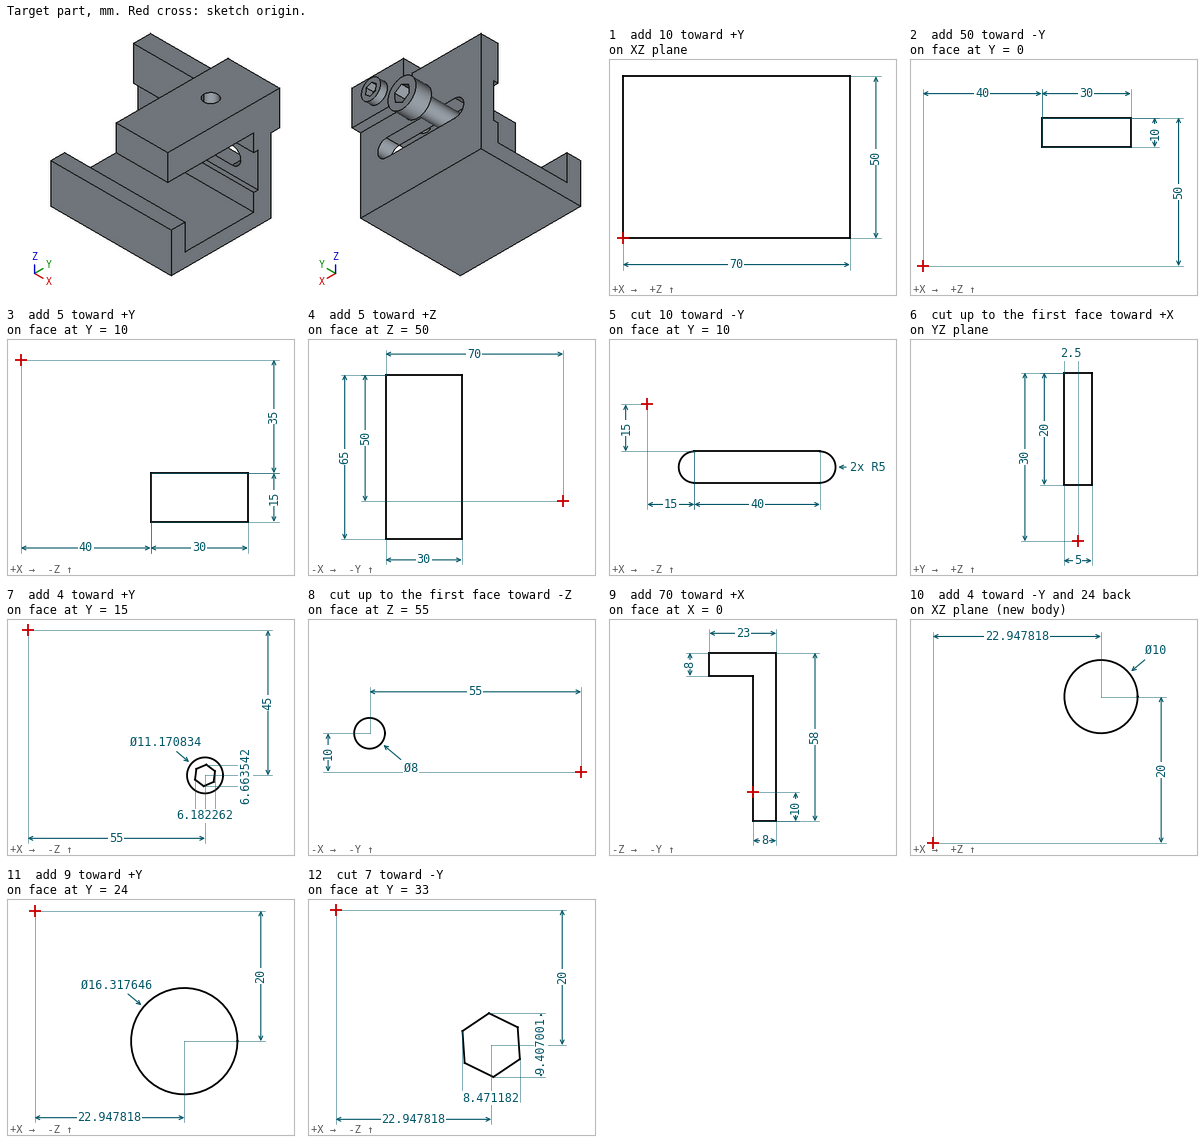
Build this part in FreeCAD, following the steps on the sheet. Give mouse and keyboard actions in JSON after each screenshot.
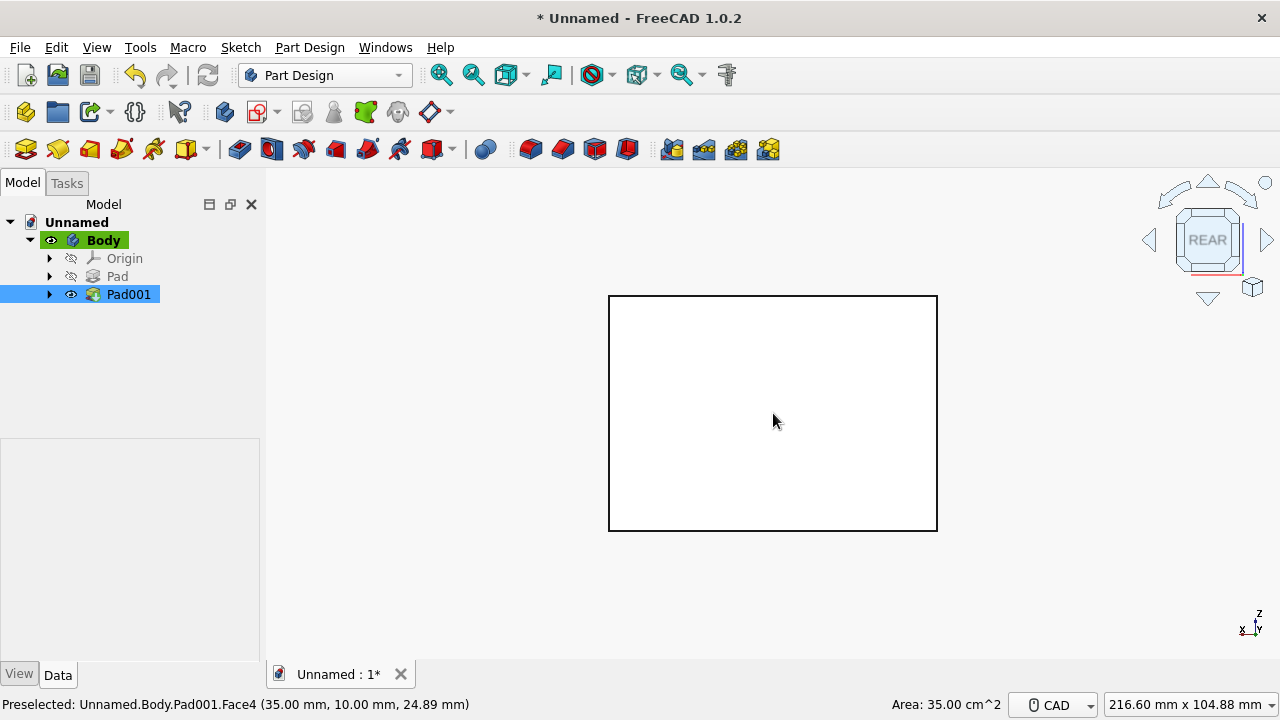
{"action": "left_click", "coordinate": [258, 112]}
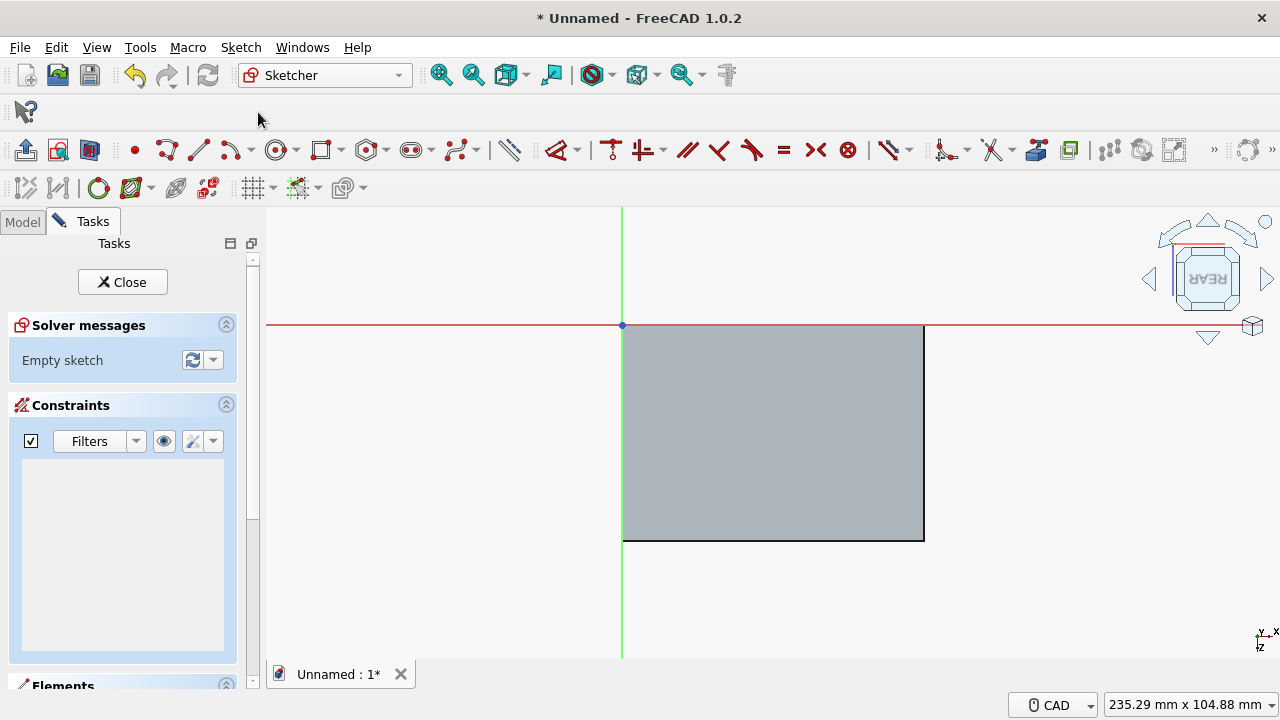
{"action": "left_click", "coordinate": [322, 150]}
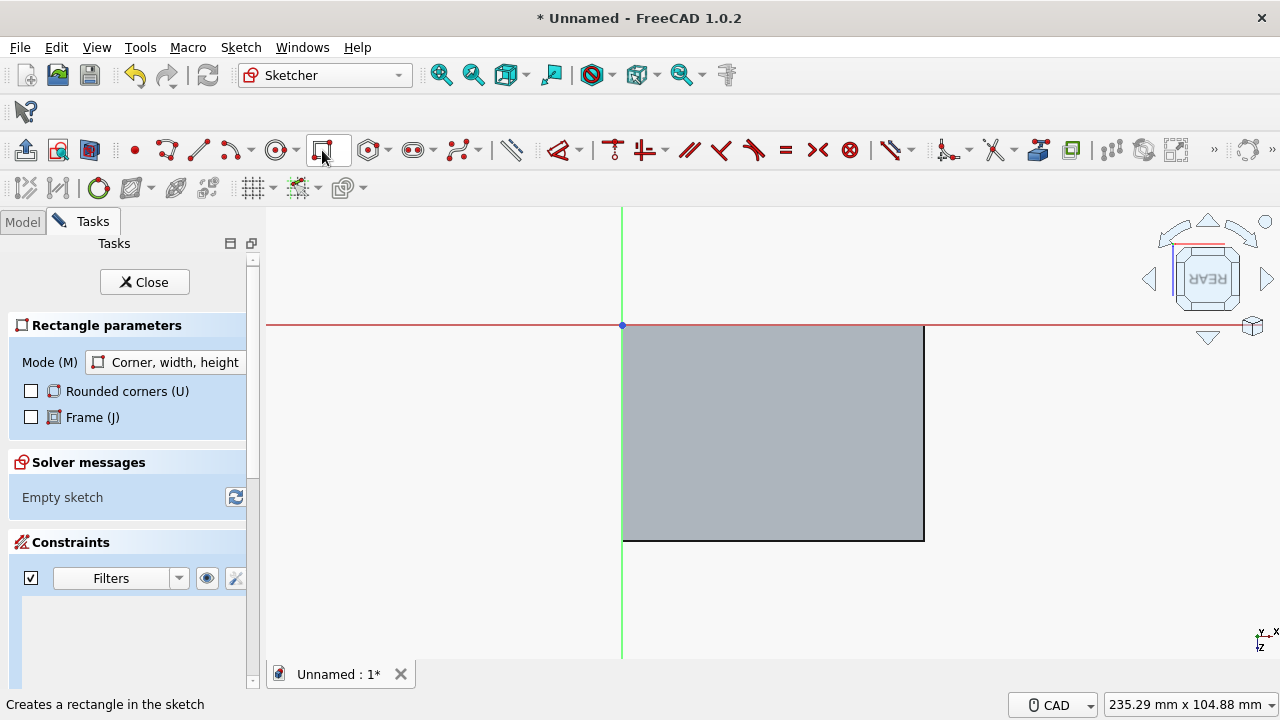
{"action": "left_click", "coordinate": [795, 476]}
{"action": "left_click", "coordinate": [924, 541]}
{"action": "key", "text": "Escape"}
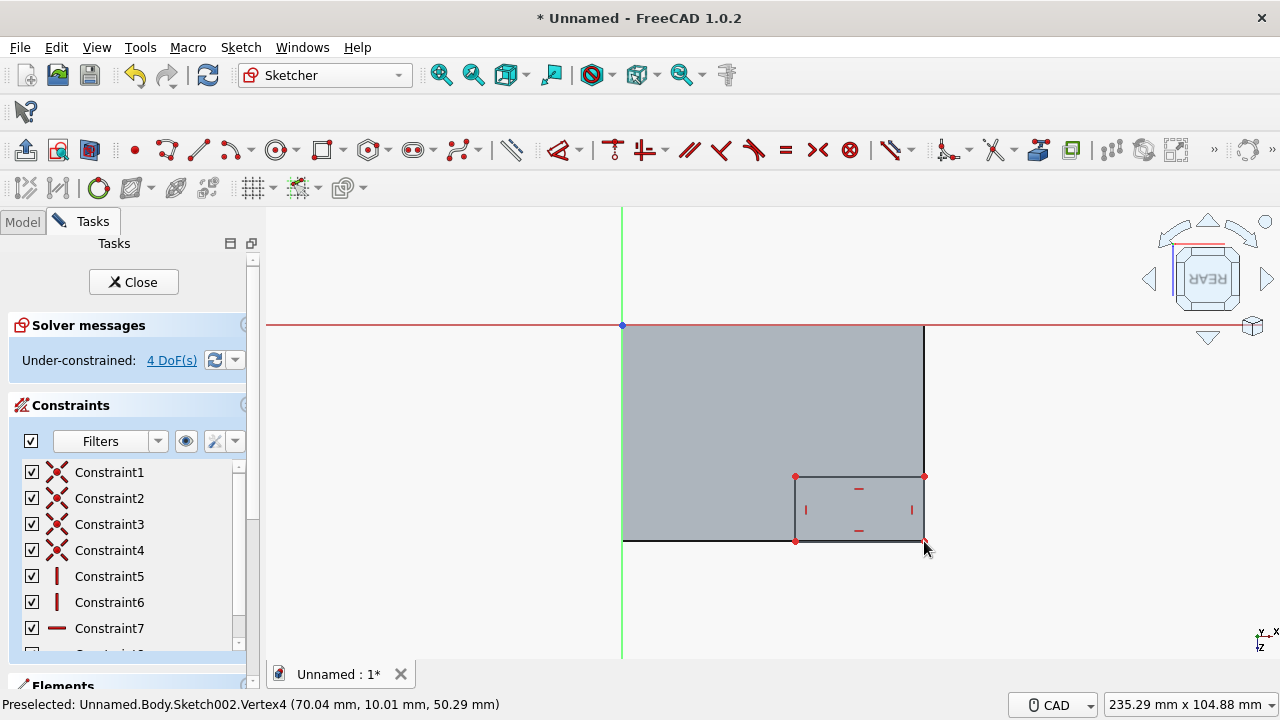
{"action": "left_click", "coordinate": [558, 150]}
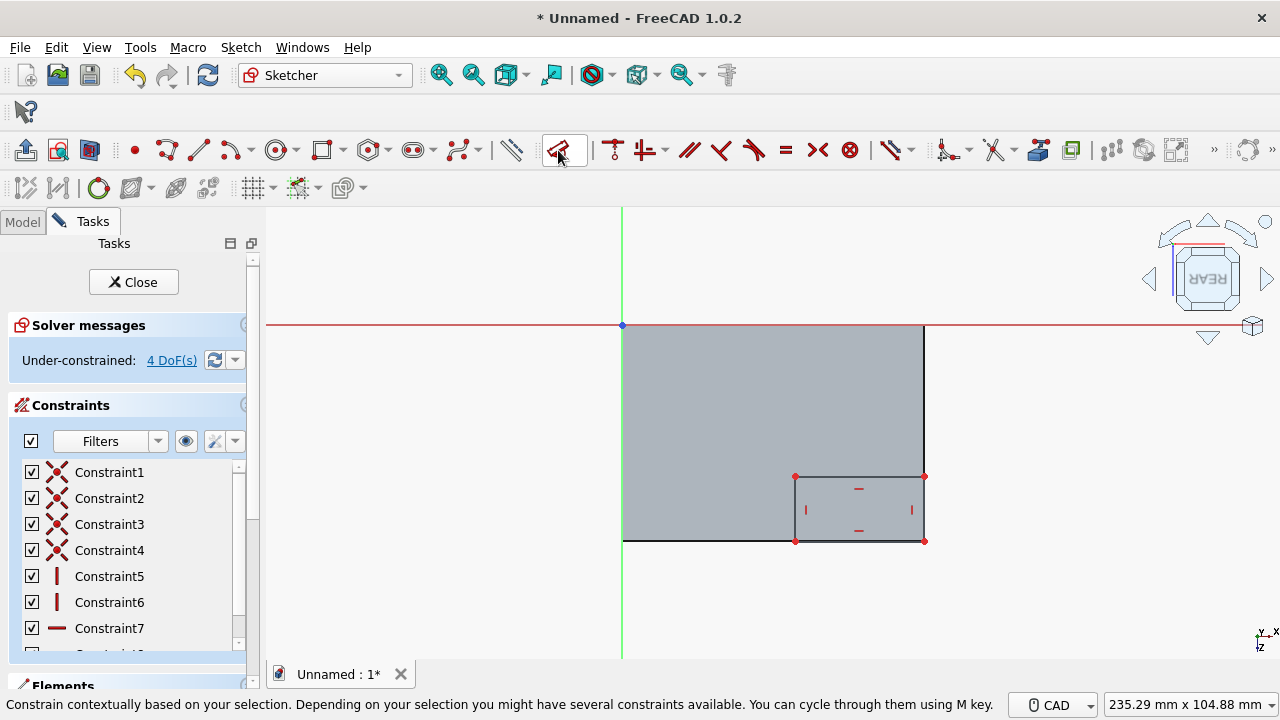
{"action": "left_click", "coordinate": [795, 497]}
{"action": "left_click", "coordinate": [829, 510]}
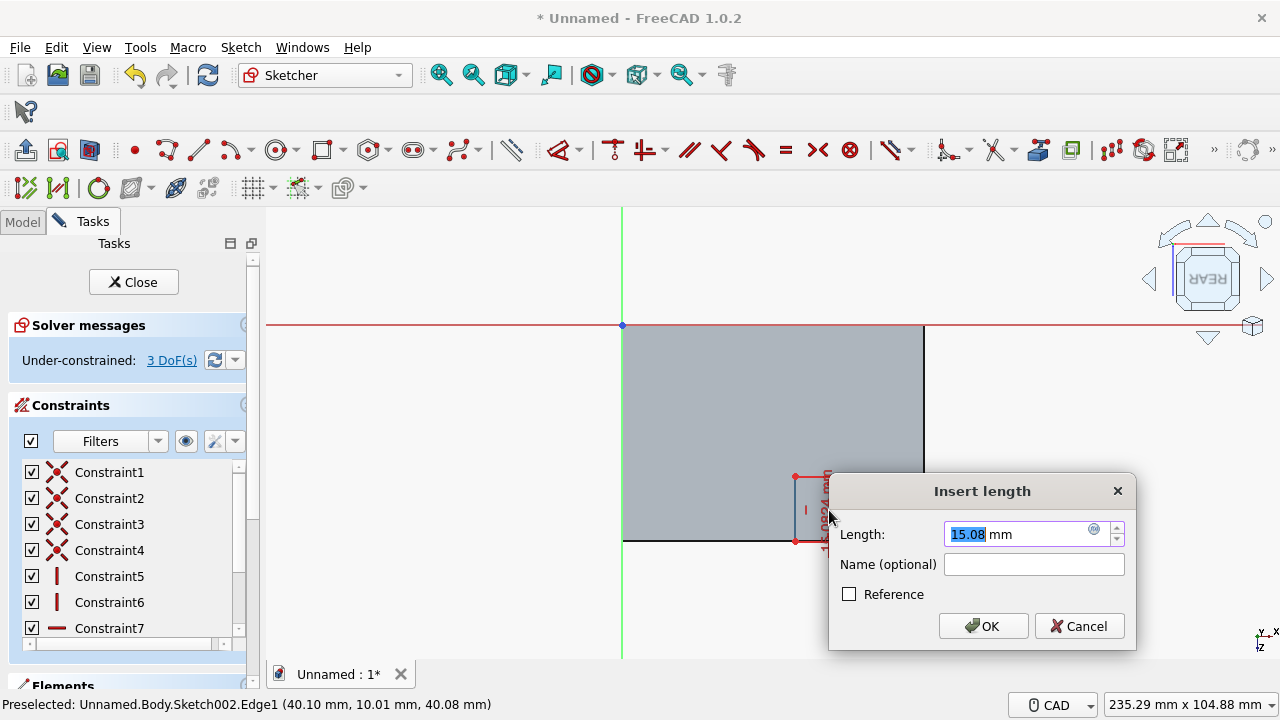
{"action": "type", "text": "15"}
{"action": "key", "text": "Return"}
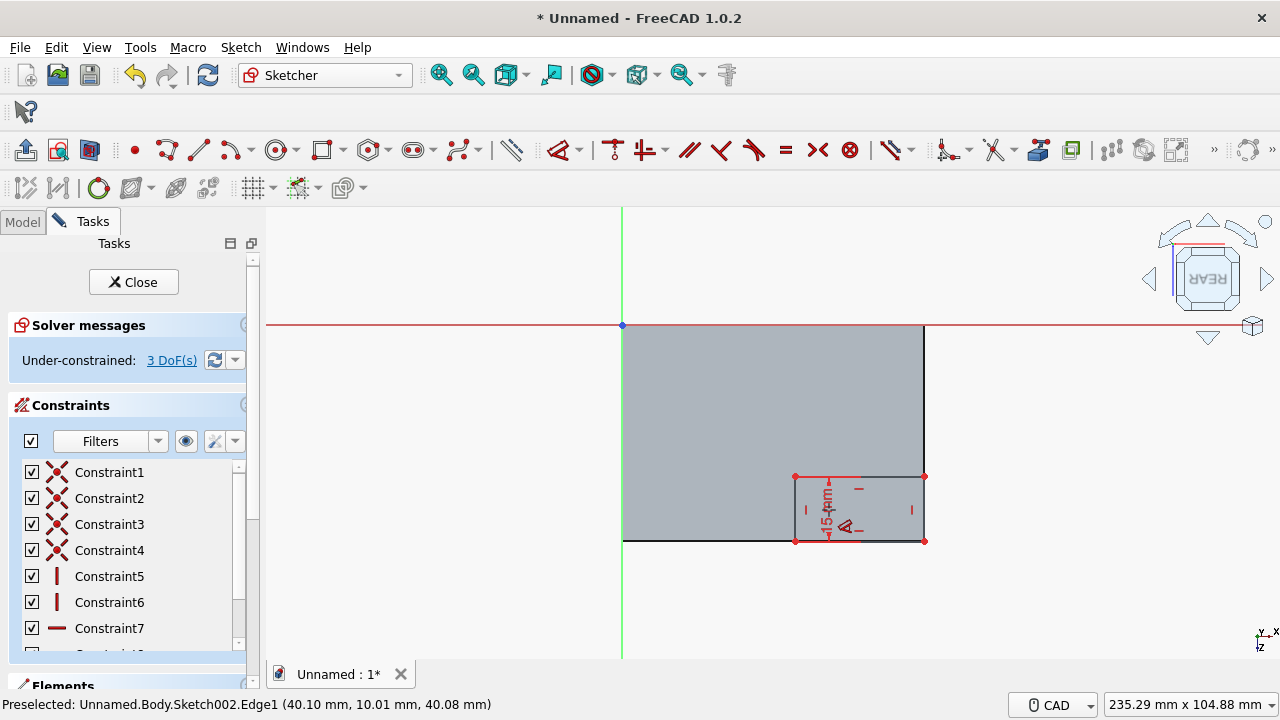
{"action": "left_click", "coordinate": [834, 542]}
{"action": "left_click", "coordinate": [860, 576]}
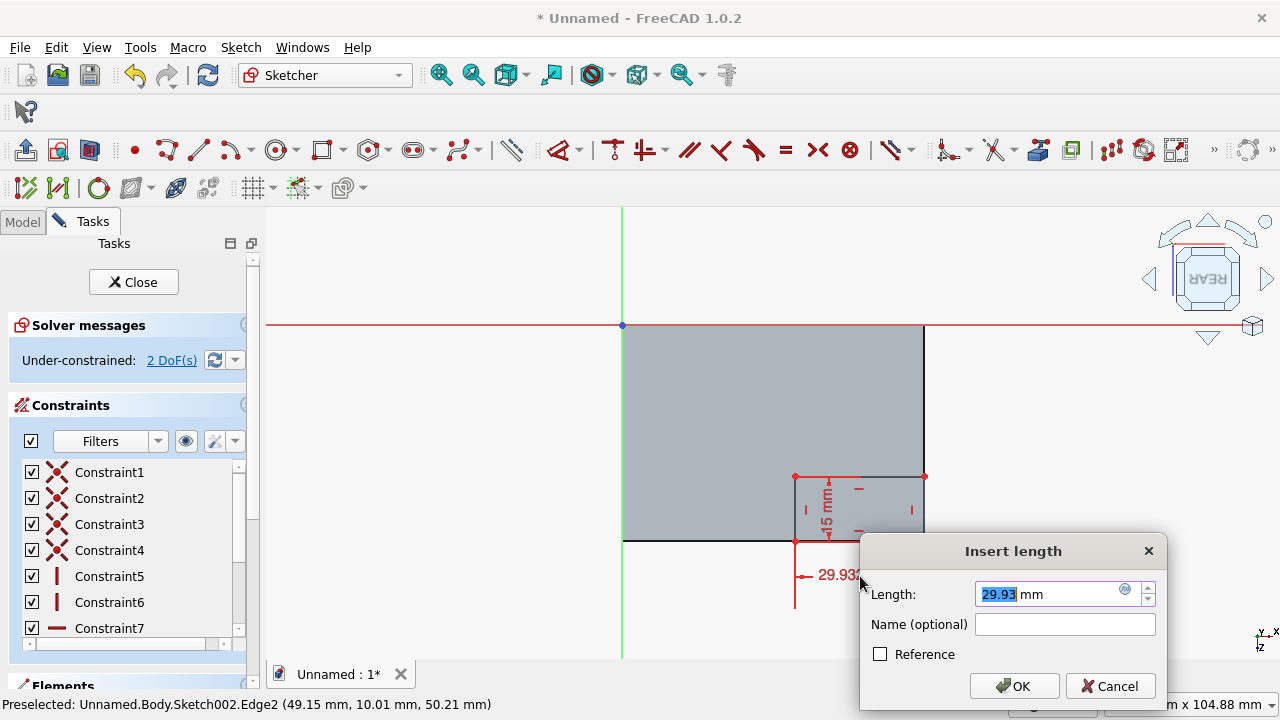
{"action": "type", "text": "30"}
{"action": "key", "text": "Return"}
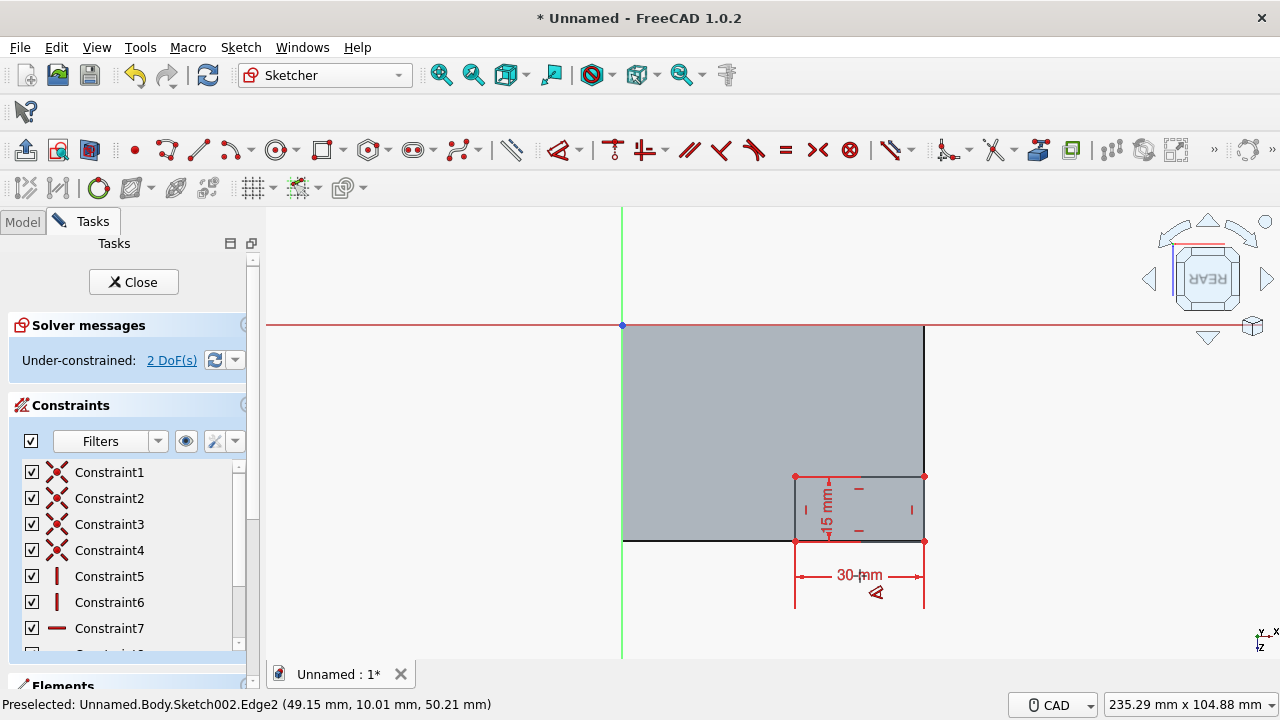
{"action": "left_click", "coordinate": [795, 477]}
{"action": "left_click", "coordinate": [709, 291]}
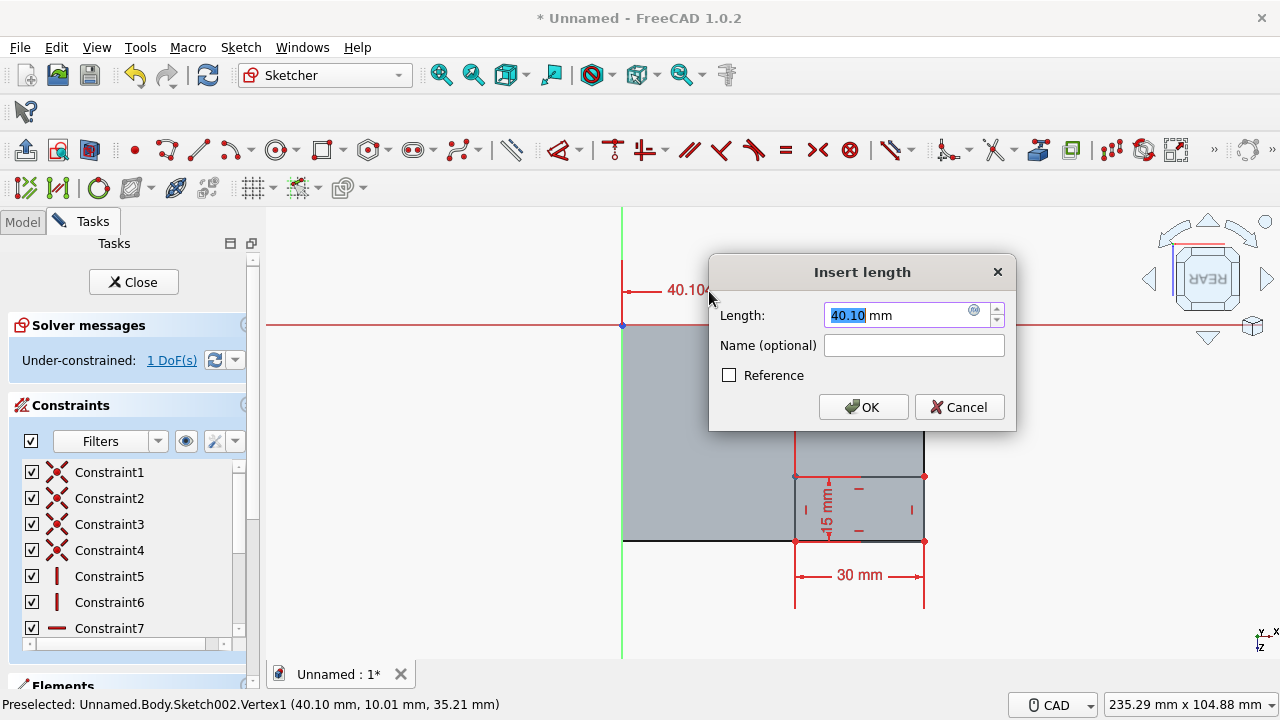
{"action": "type", "text": "40"}
{"action": "key", "text": "Return"}